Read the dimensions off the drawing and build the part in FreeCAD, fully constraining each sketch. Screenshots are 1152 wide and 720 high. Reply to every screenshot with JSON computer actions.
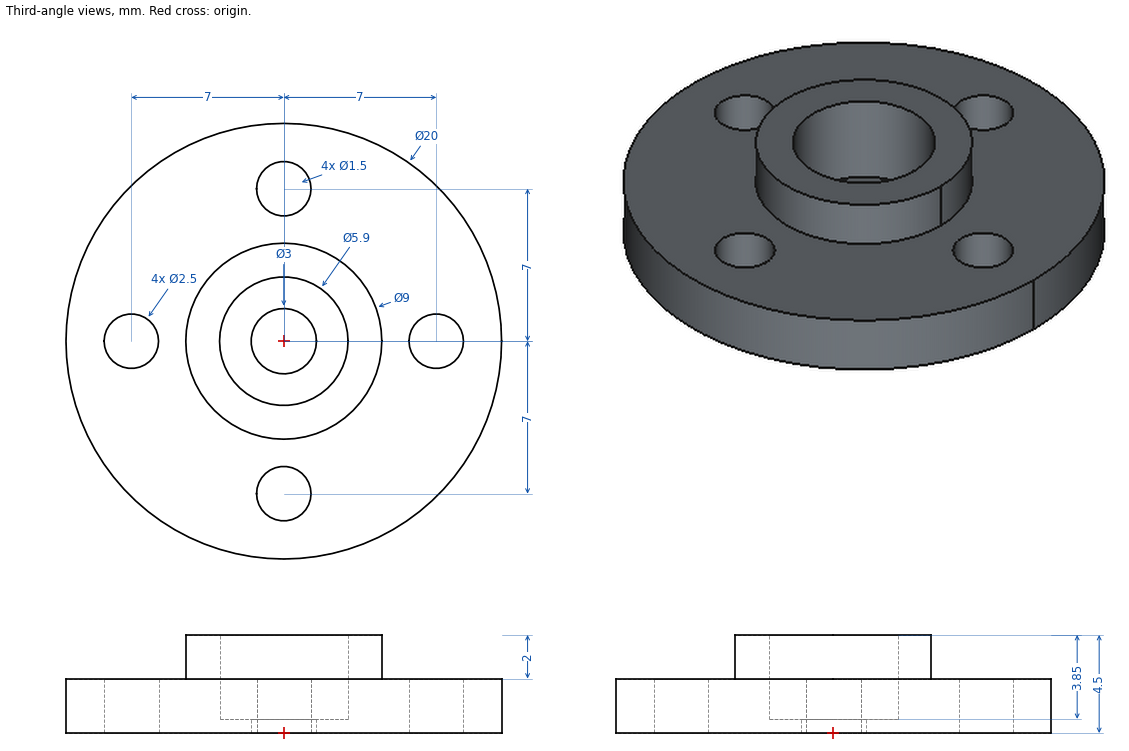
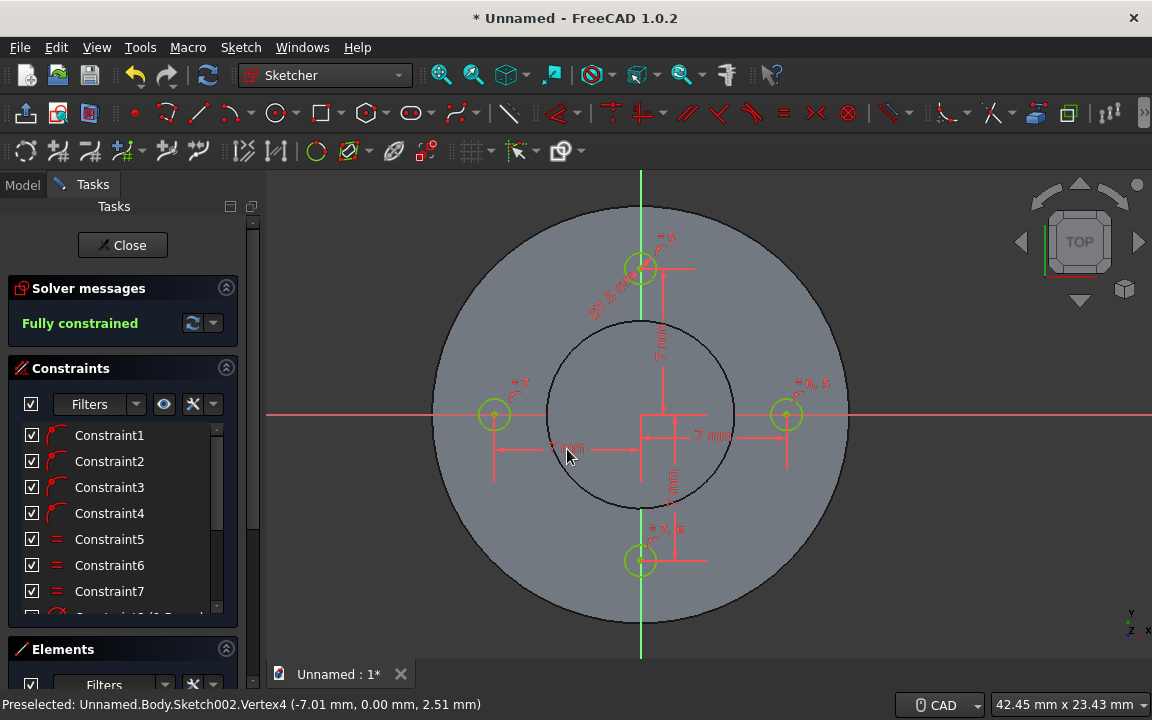
{"action": "left_click", "coordinate": [123, 245]}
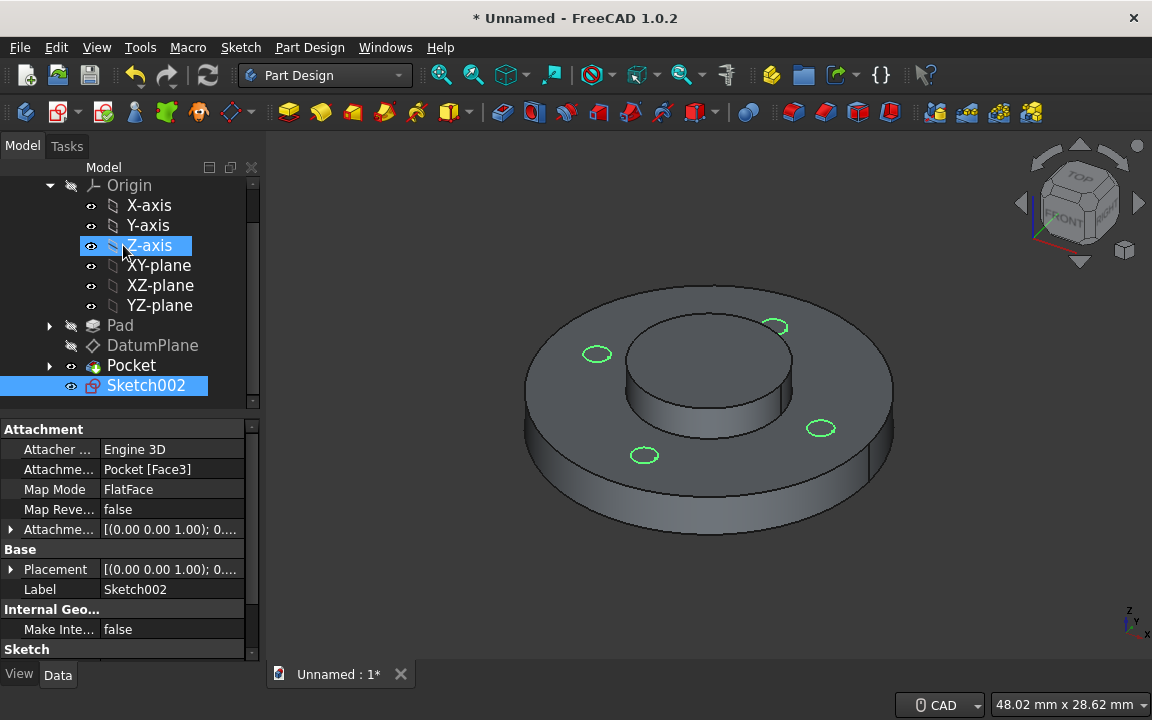
{"action": "left_click", "coordinate": [504, 112]}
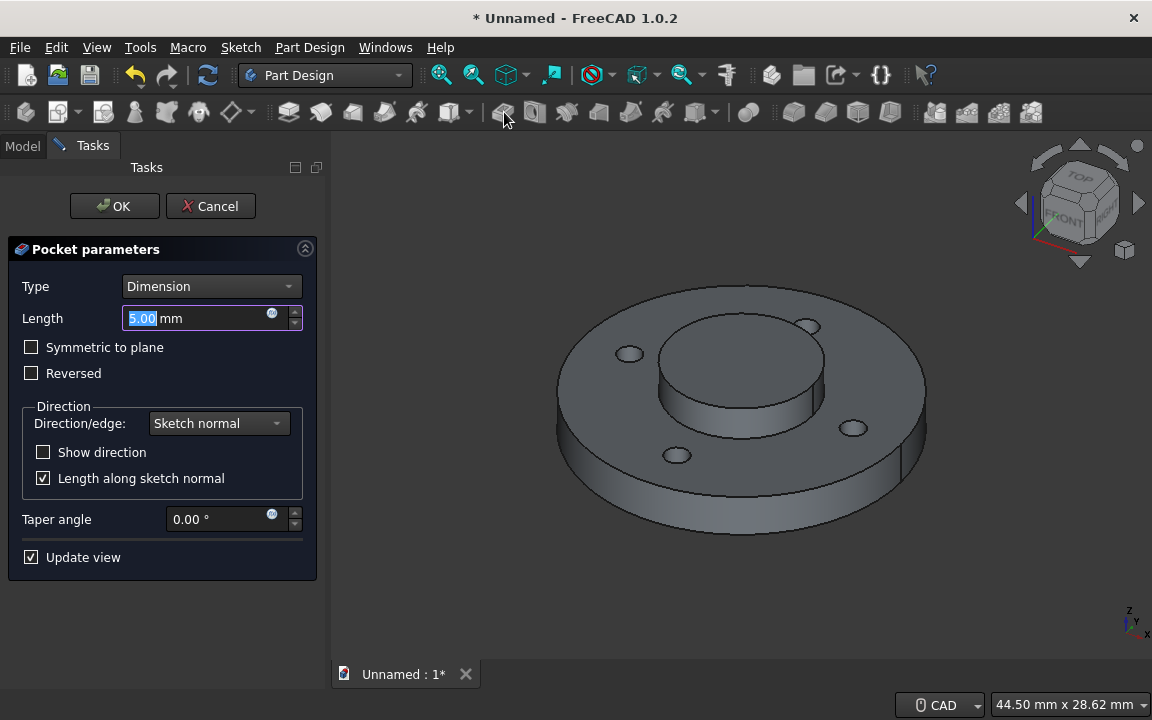
{"action": "left_click", "coordinate": [212, 286]}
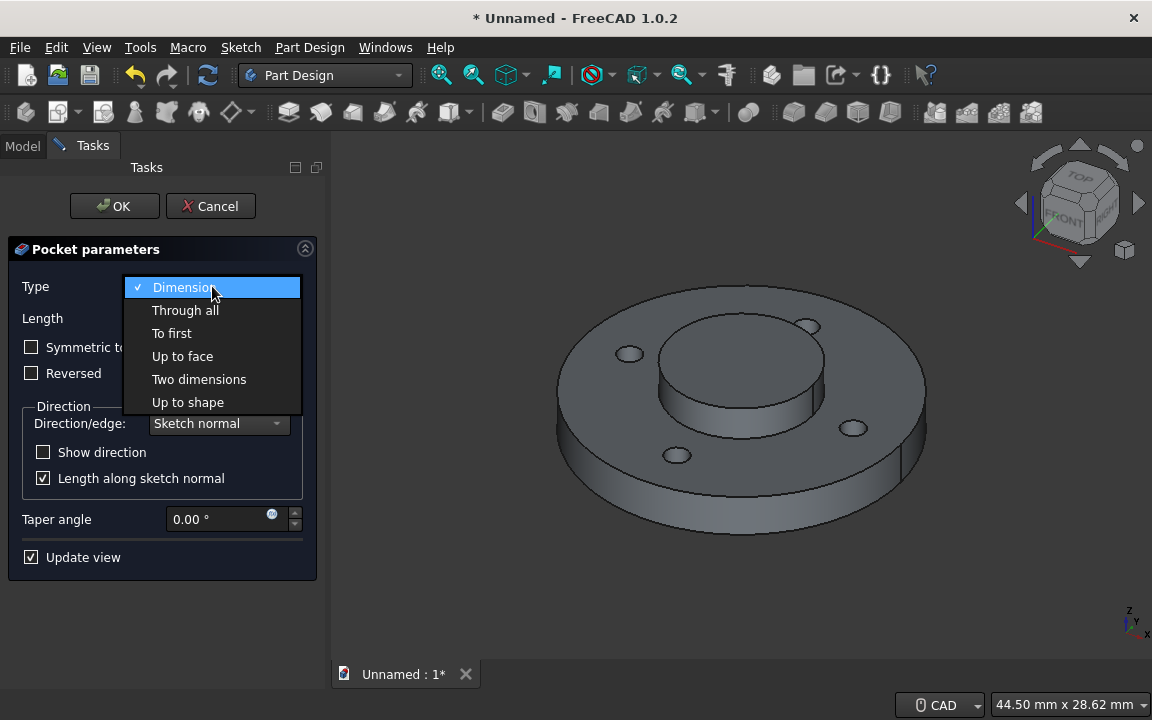
{"action": "left_click", "coordinate": [212, 310]}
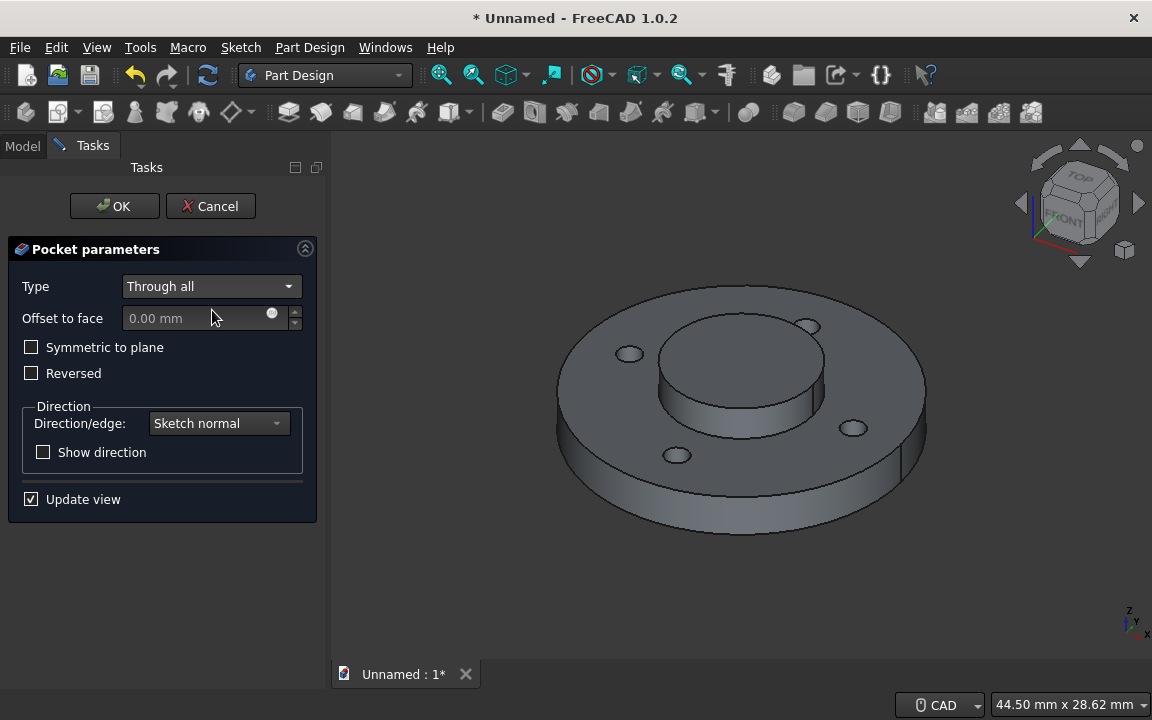
{"action": "left_click", "coordinate": [115, 206]}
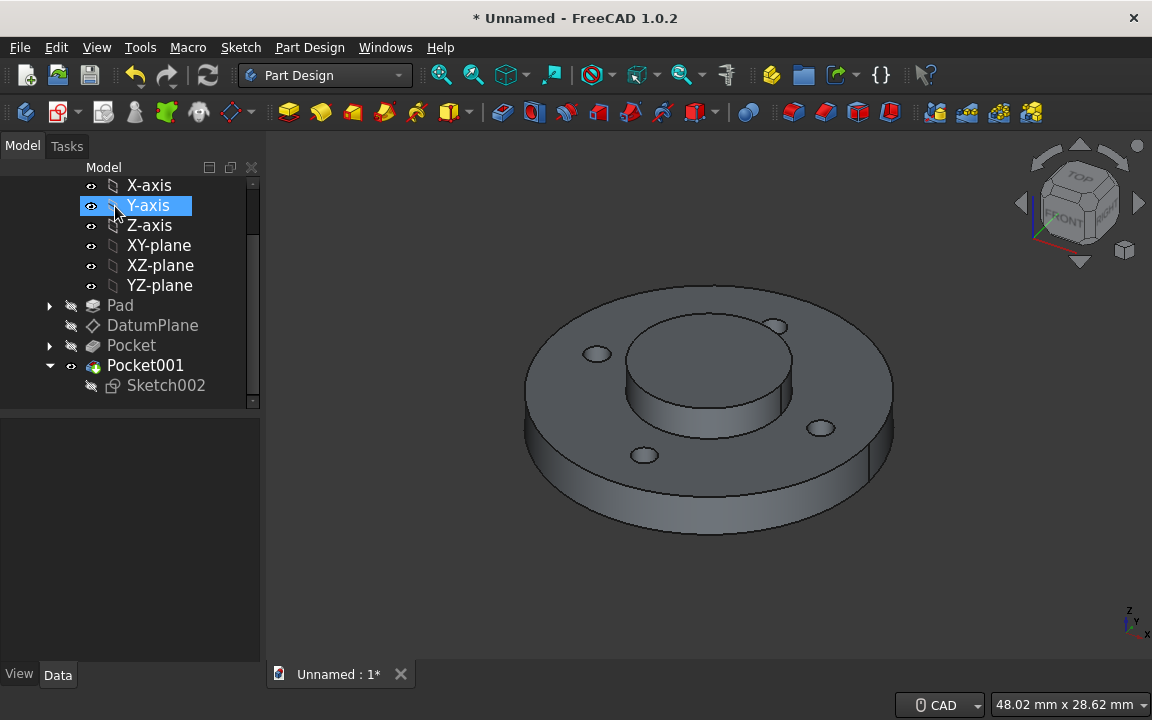
{"action": "left_click", "coordinate": [709, 360]}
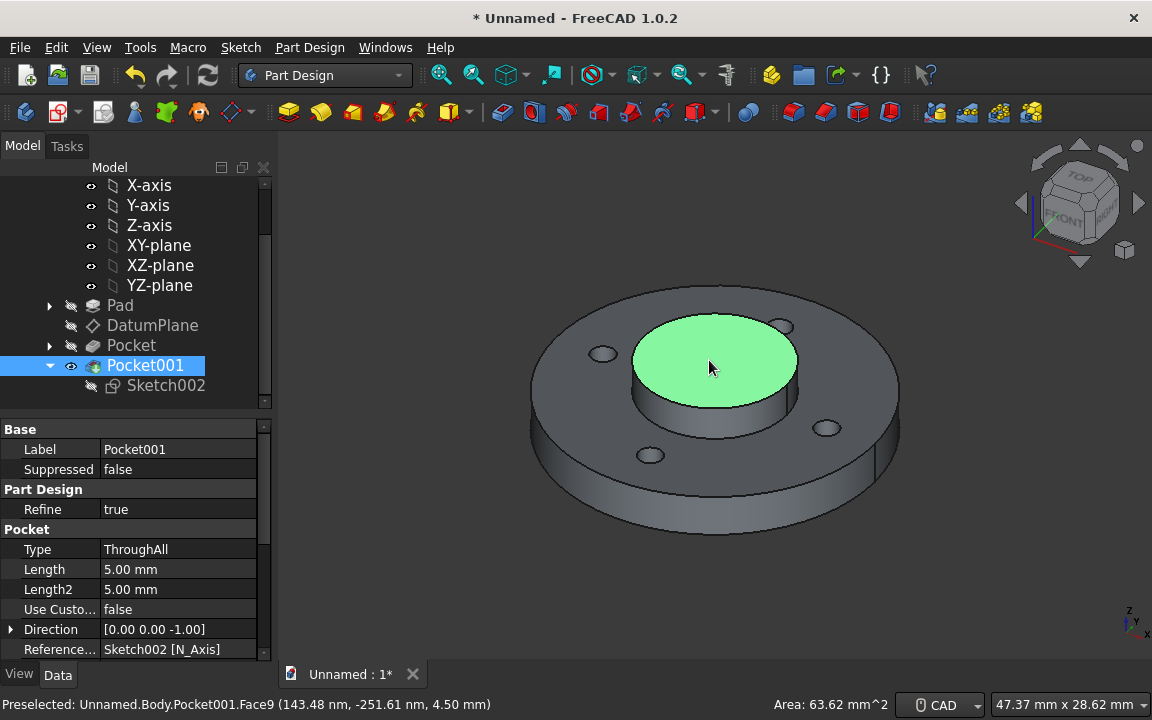
{"action": "left_click", "coordinate": [58, 112]}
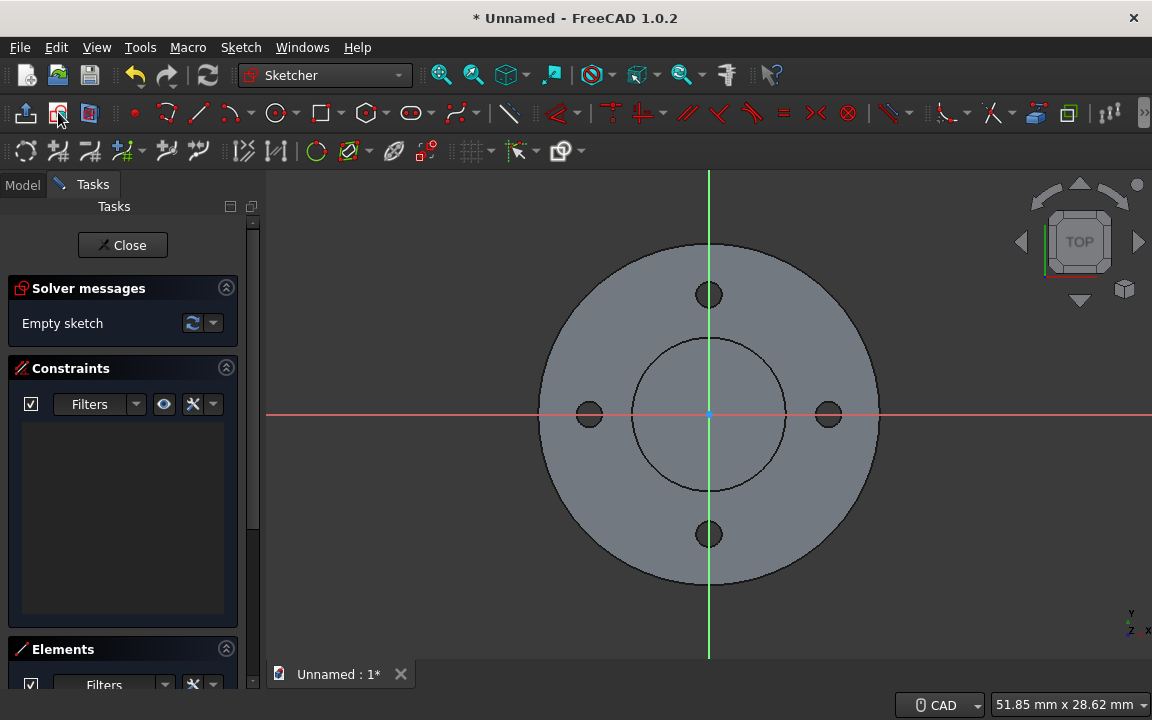
{"action": "scroll", "coordinate": [739, 415], "scroll_direction": "up", "scroll_amount": 6}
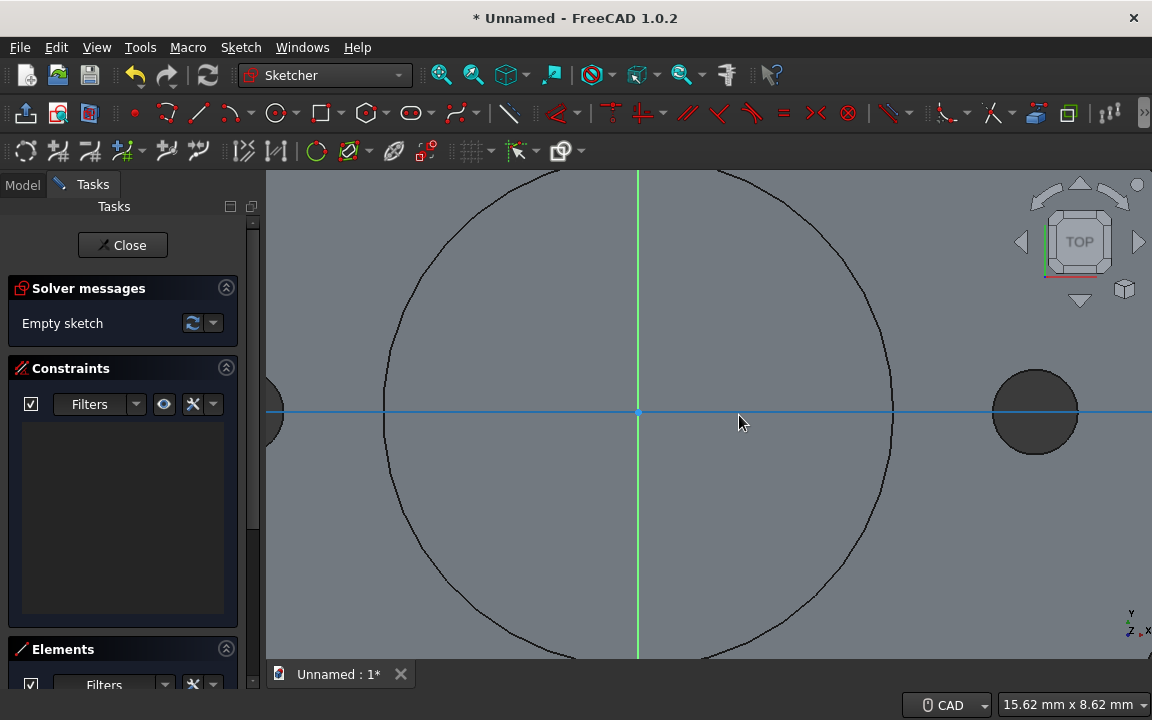
{"action": "left_click", "coordinate": [276, 114]}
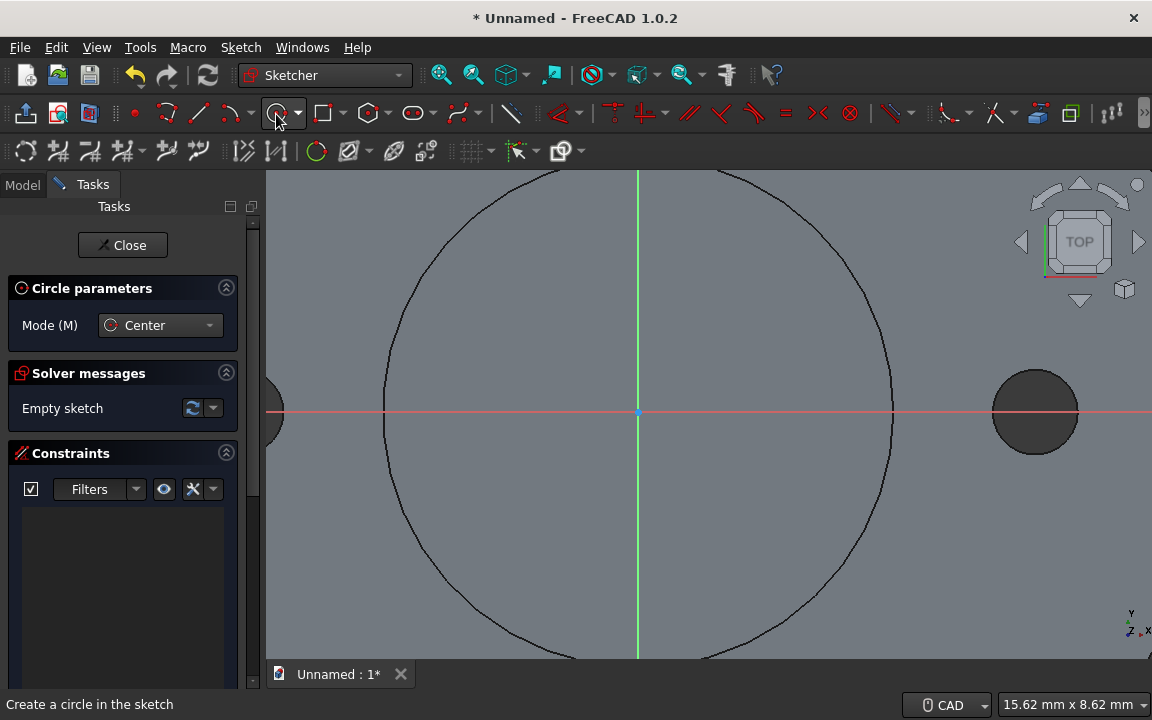
{"action": "left_click", "coordinate": [638, 412]}
{"action": "left_click", "coordinate": [756, 294]}
{"action": "key", "text": "Escape"}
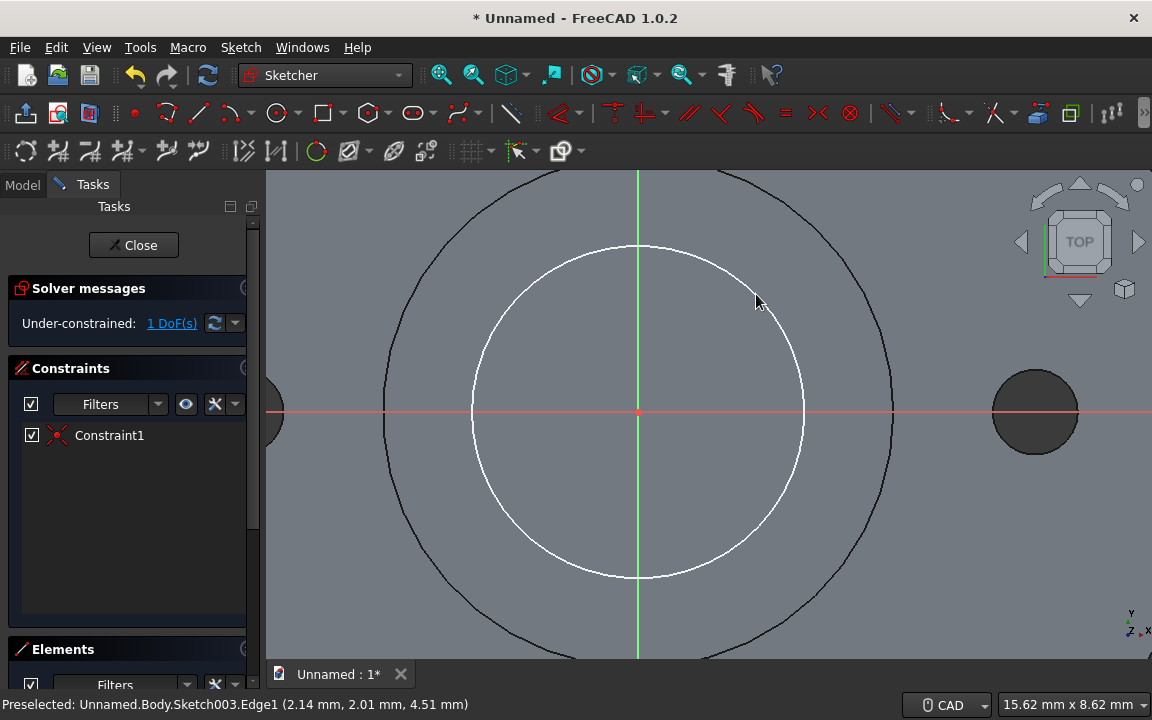
{"action": "key", "text": "d"}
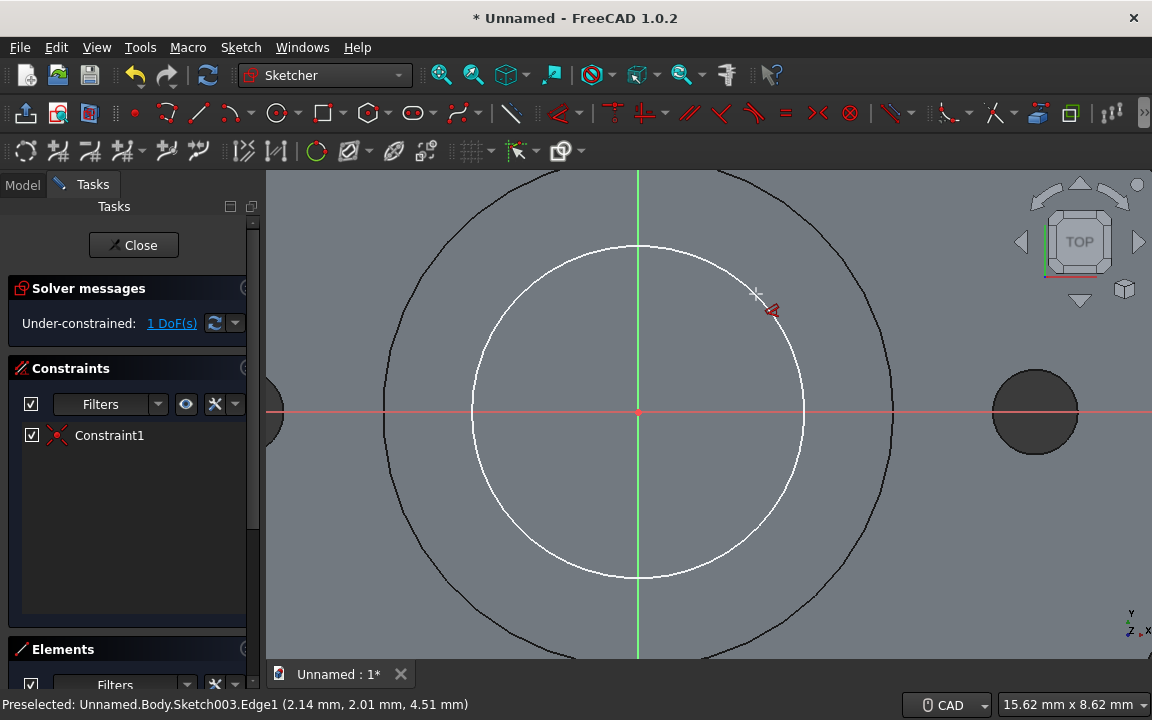
{"action": "left_click", "coordinate": [755, 294]}
{"action": "left_click", "coordinate": [777, 271]}